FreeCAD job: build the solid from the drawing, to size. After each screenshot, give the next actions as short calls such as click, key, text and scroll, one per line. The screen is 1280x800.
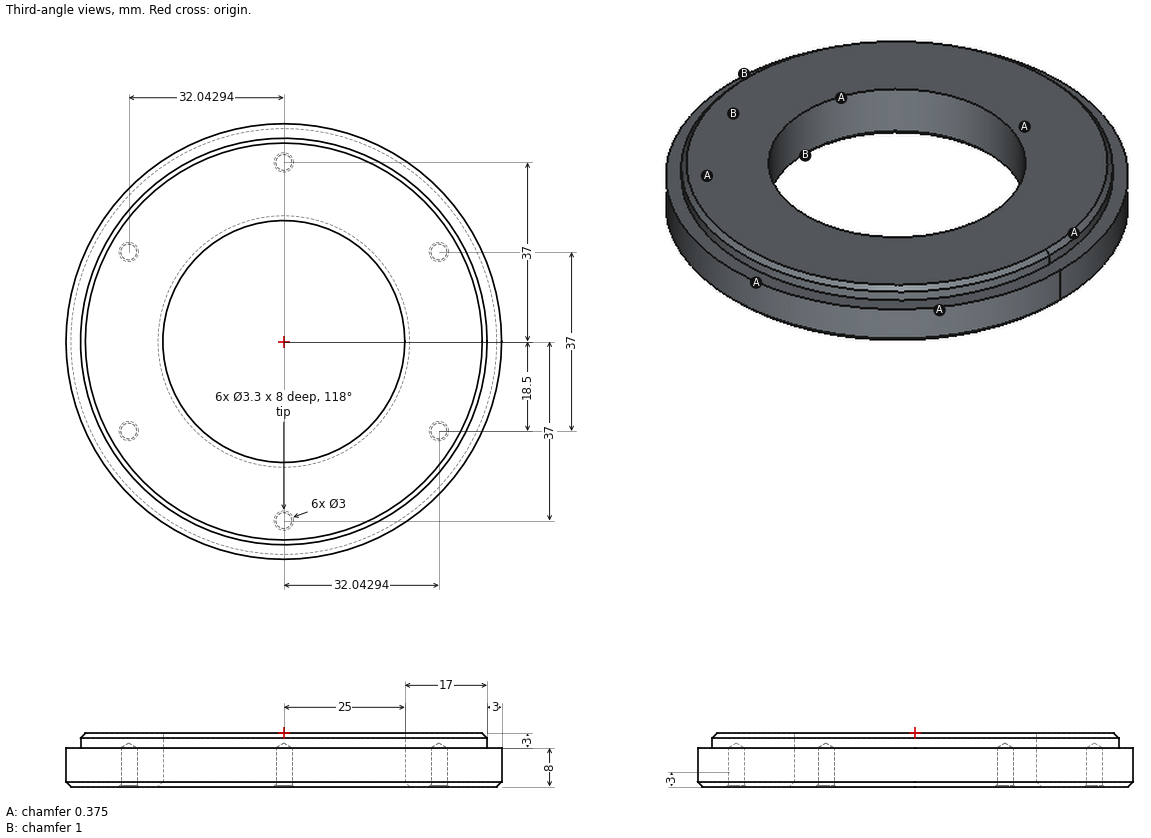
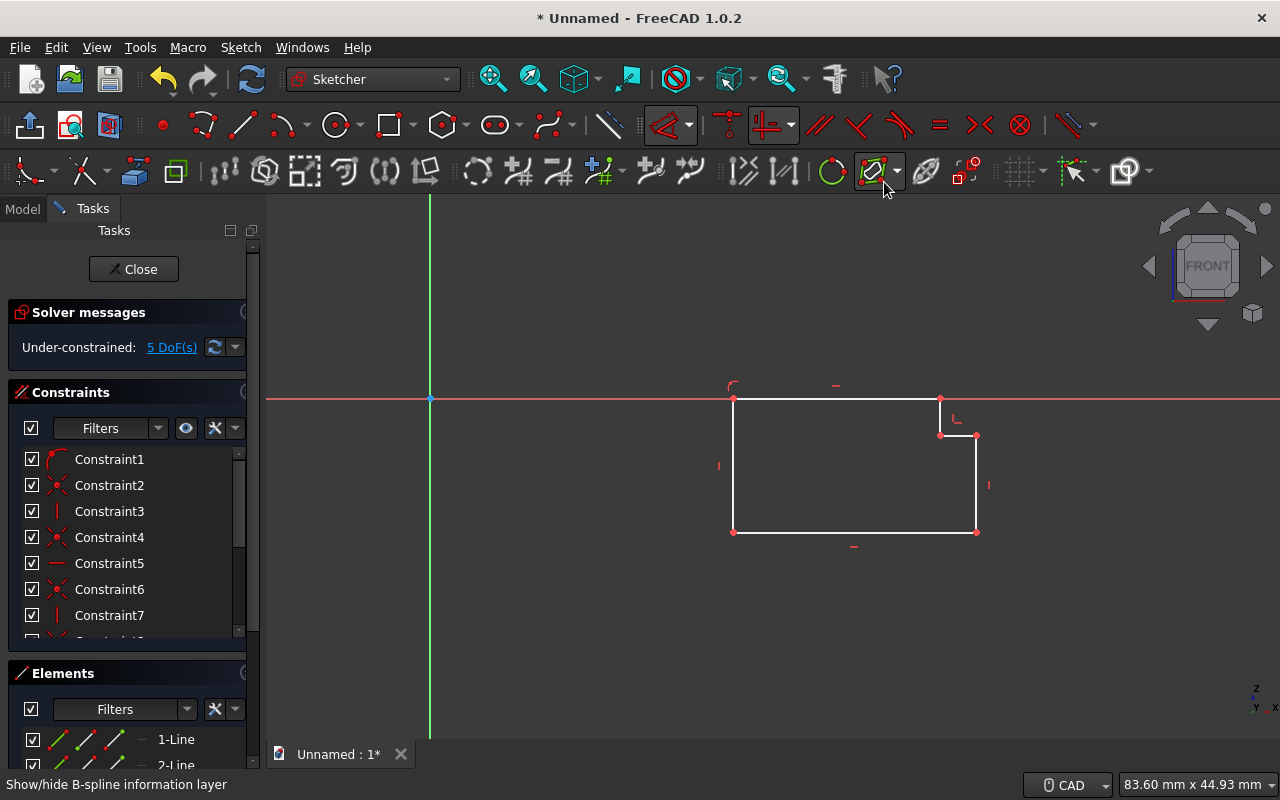
click(664, 126)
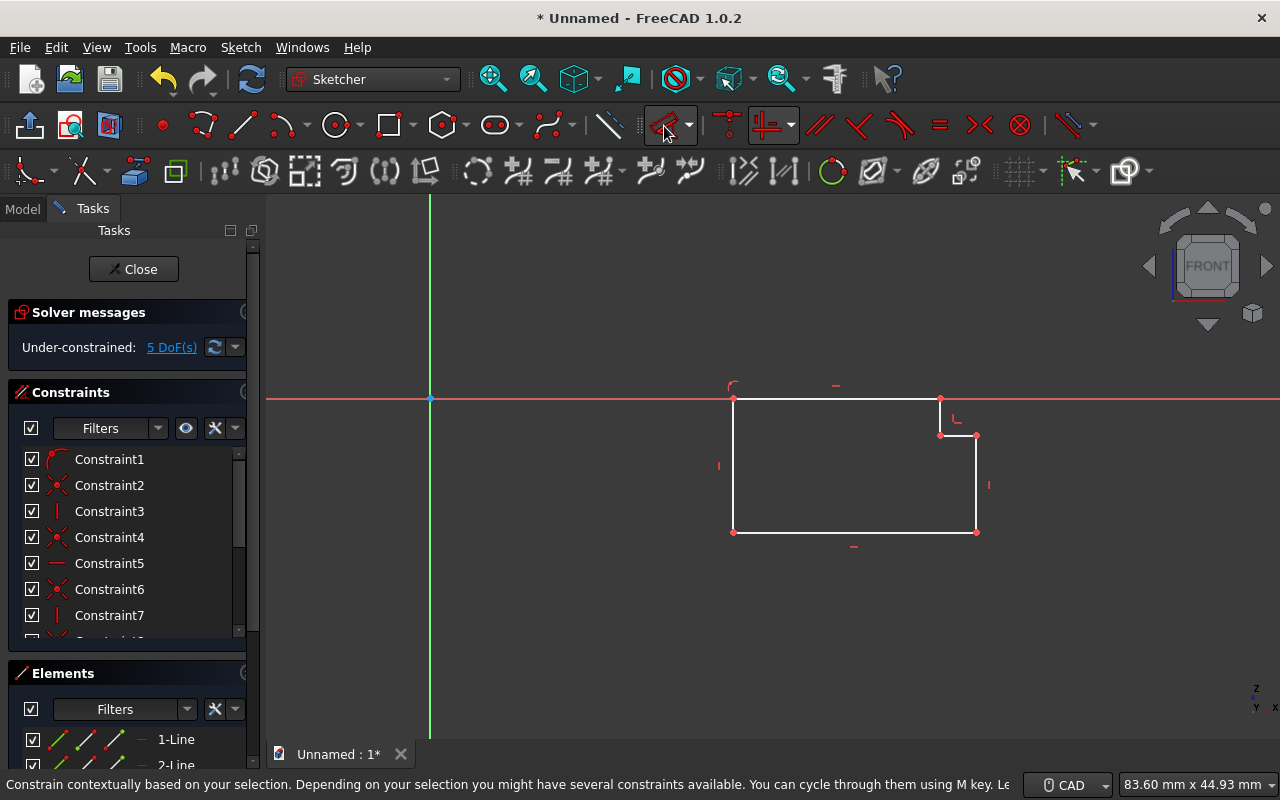
scroll(940, 410, up, 2)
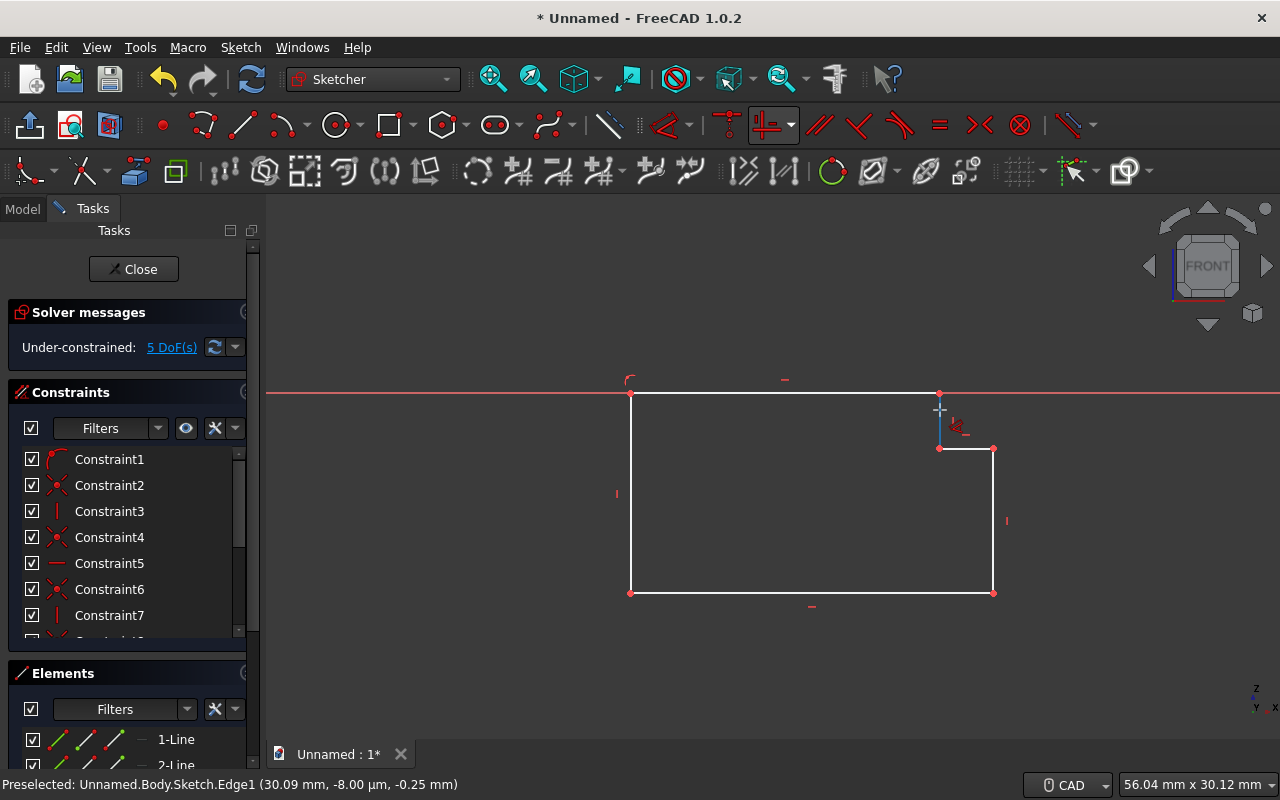
click(940, 410)
click(974, 421)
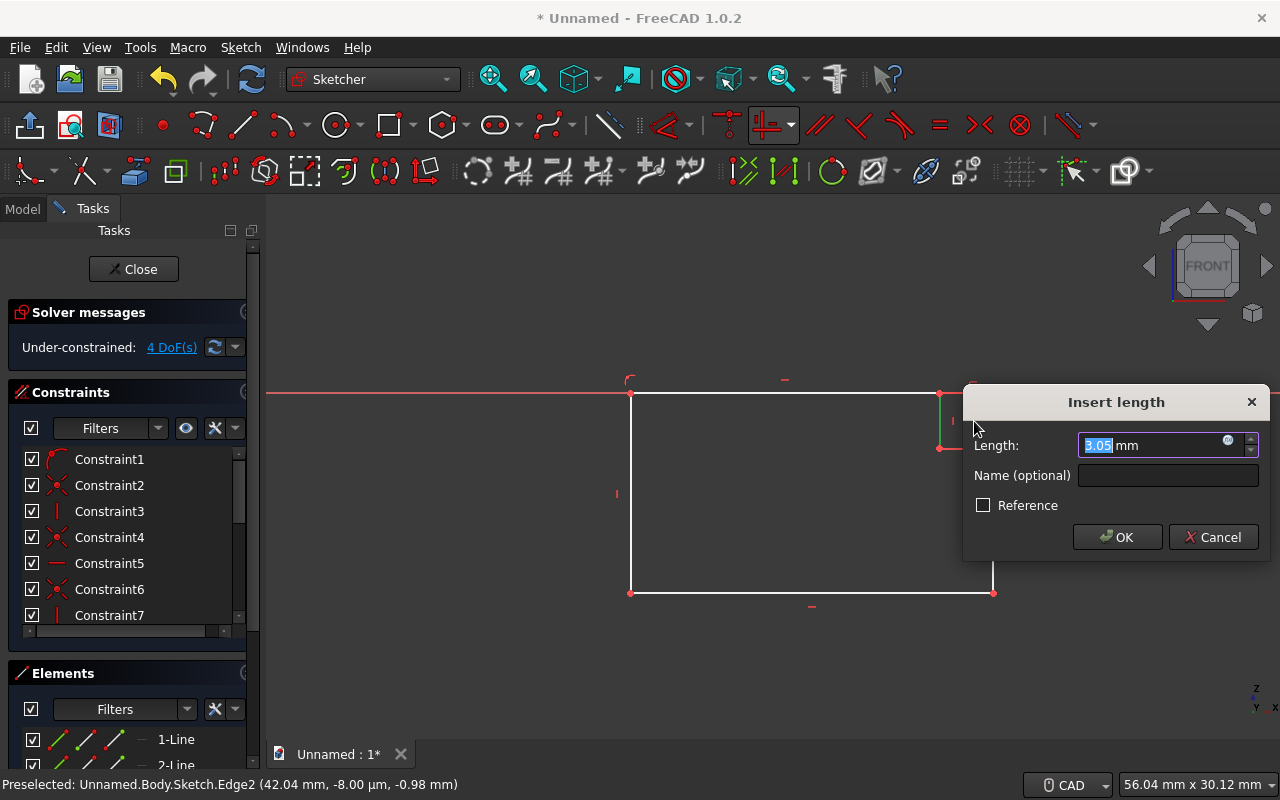
text(3)
key(Return)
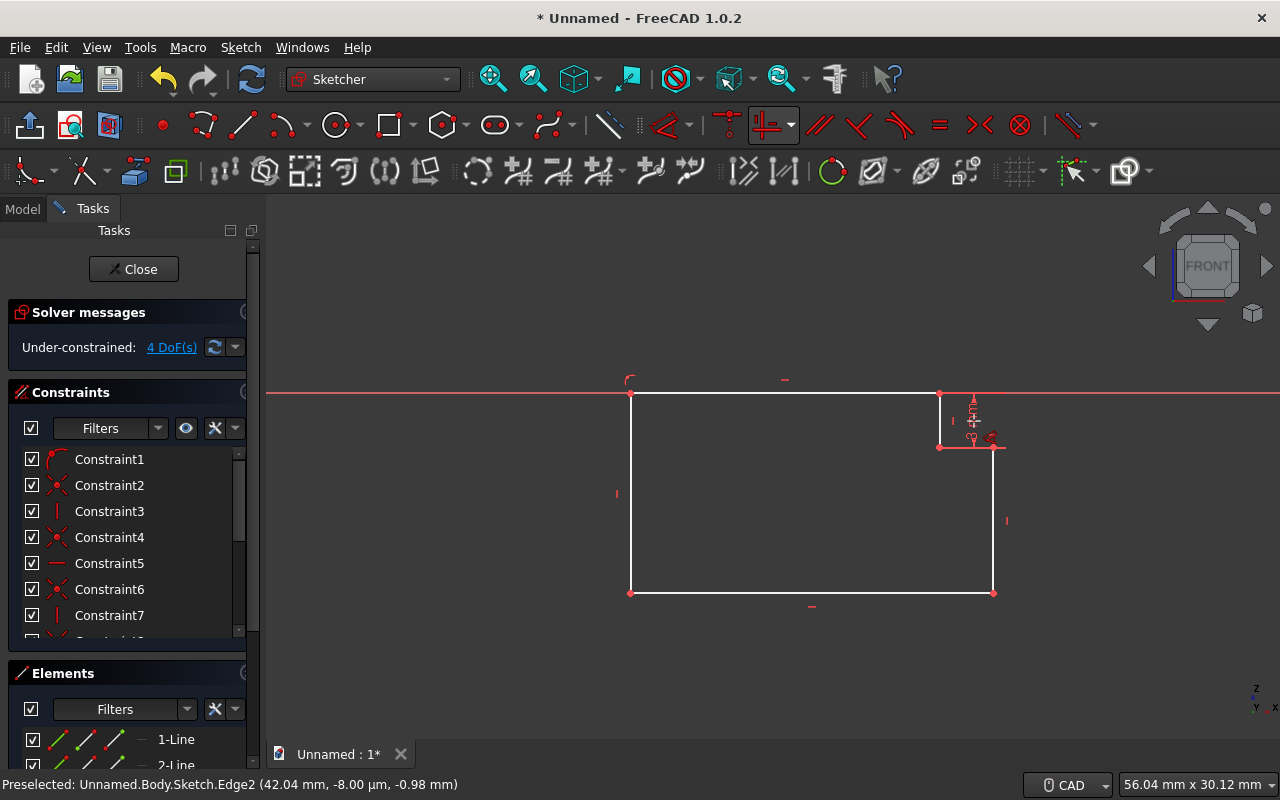
click(956, 448)
click(967, 482)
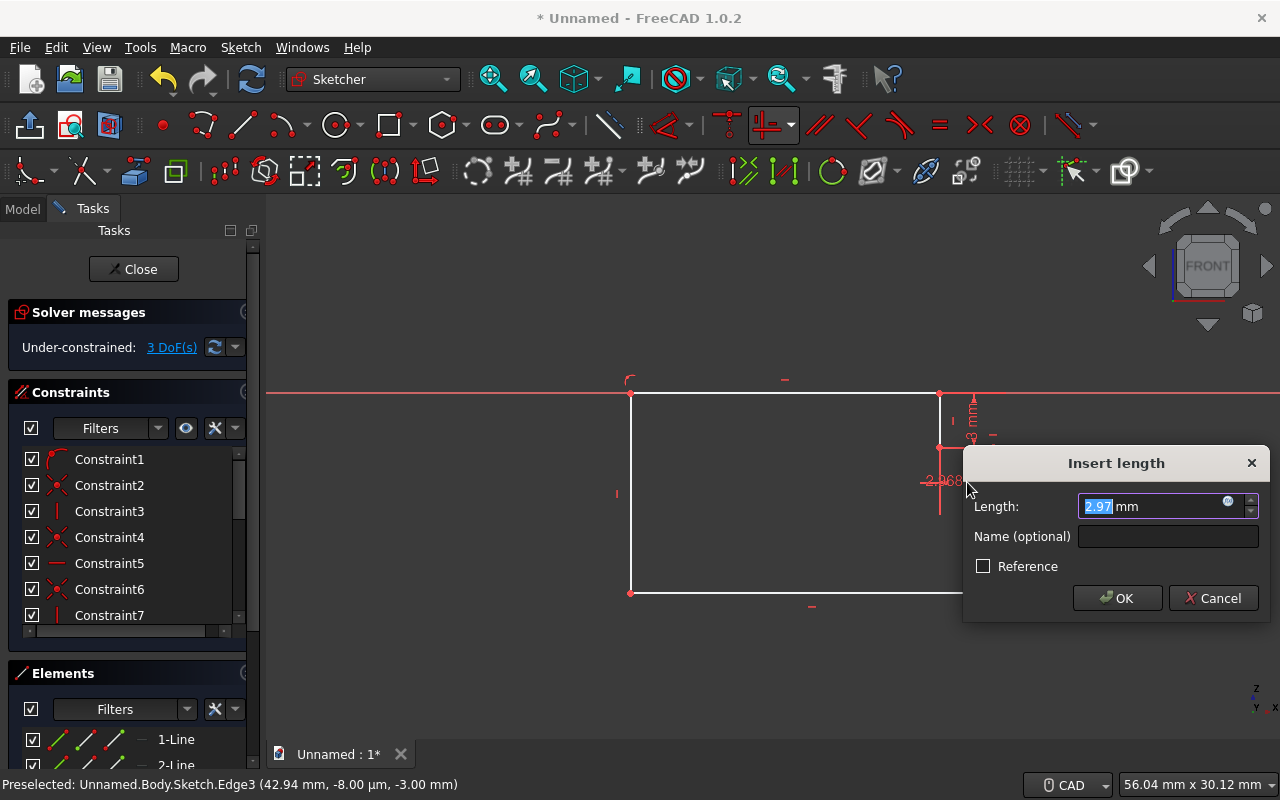
text(3)
key(Return)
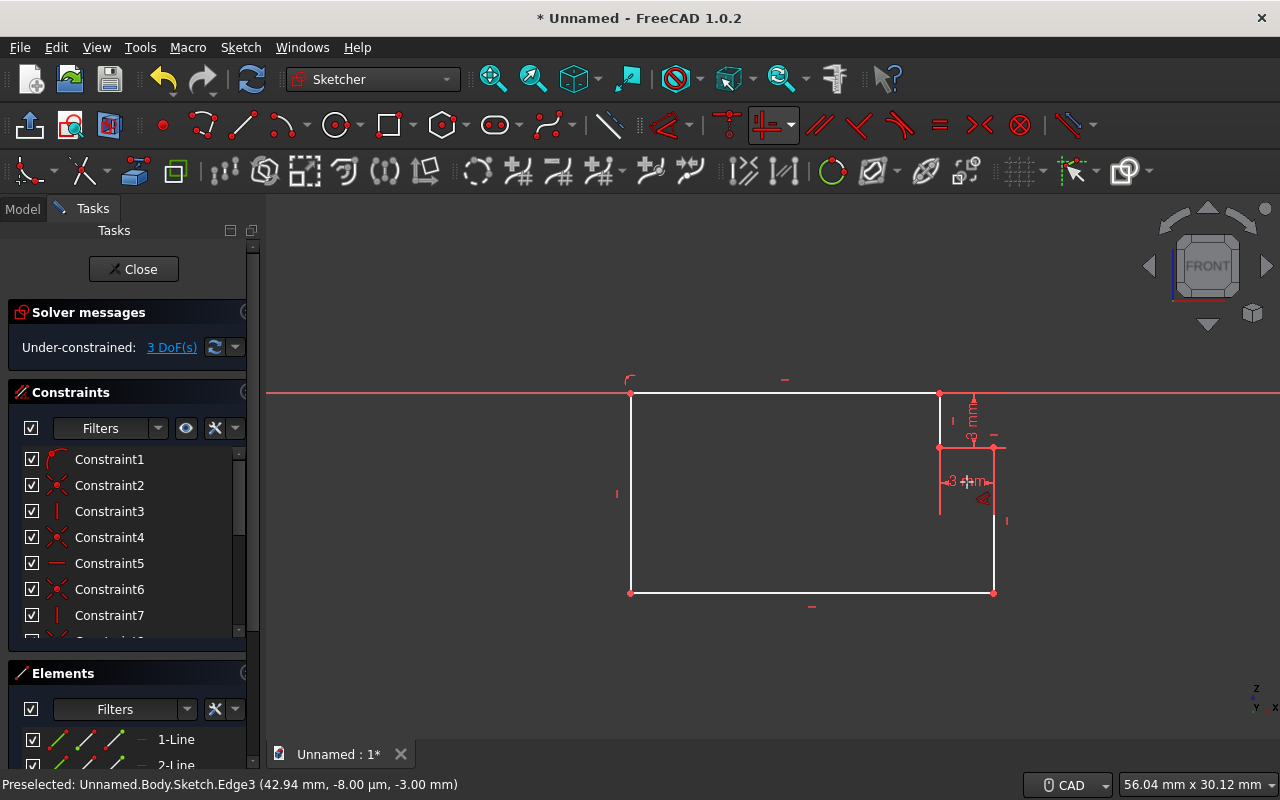
click(994, 491)
click(1028, 520)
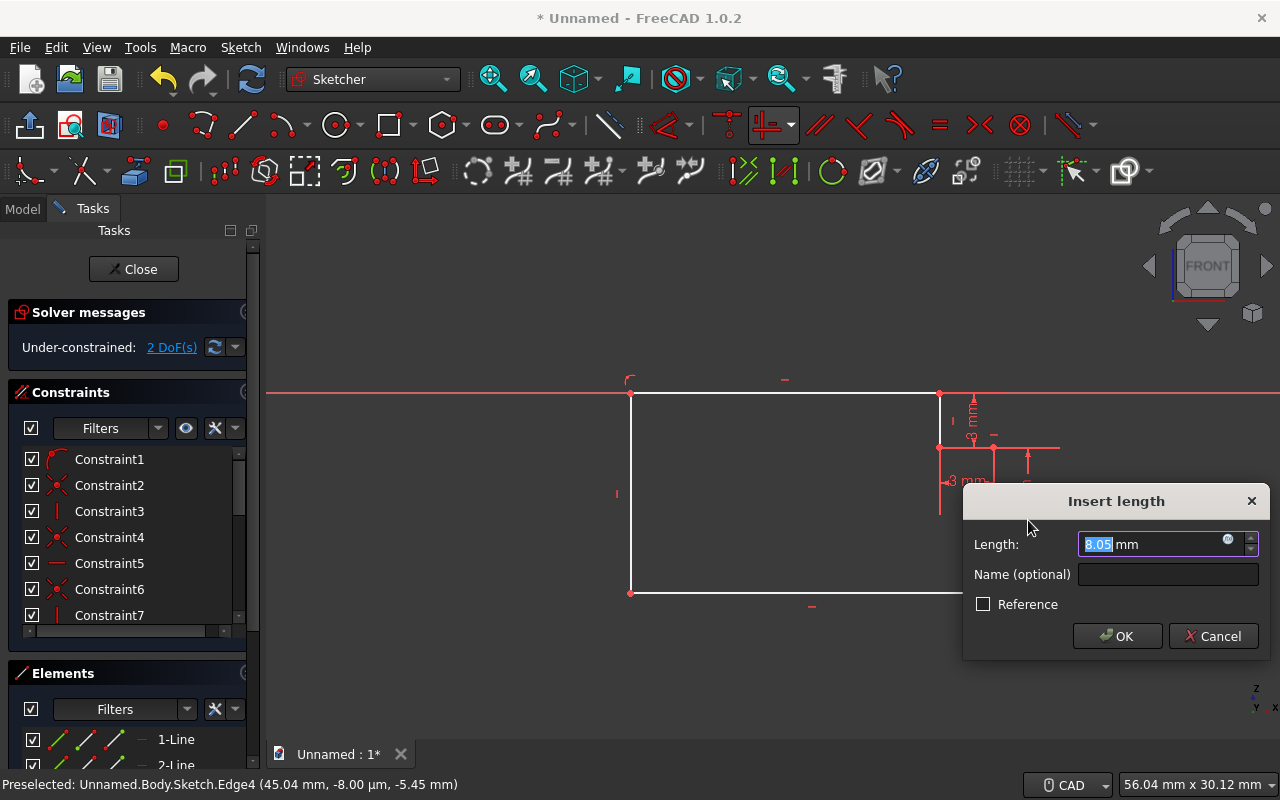
text(8)
key(Return)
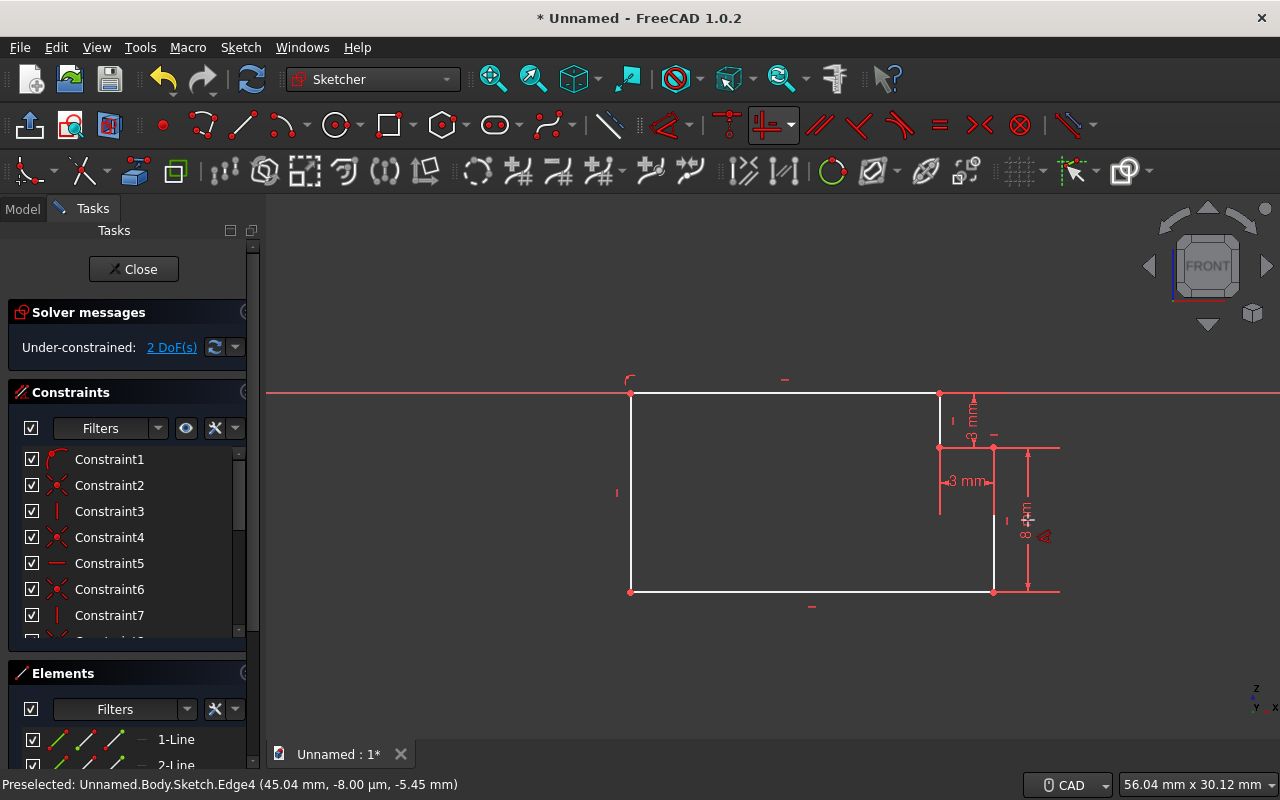
click(724, 393)
click(785, 359)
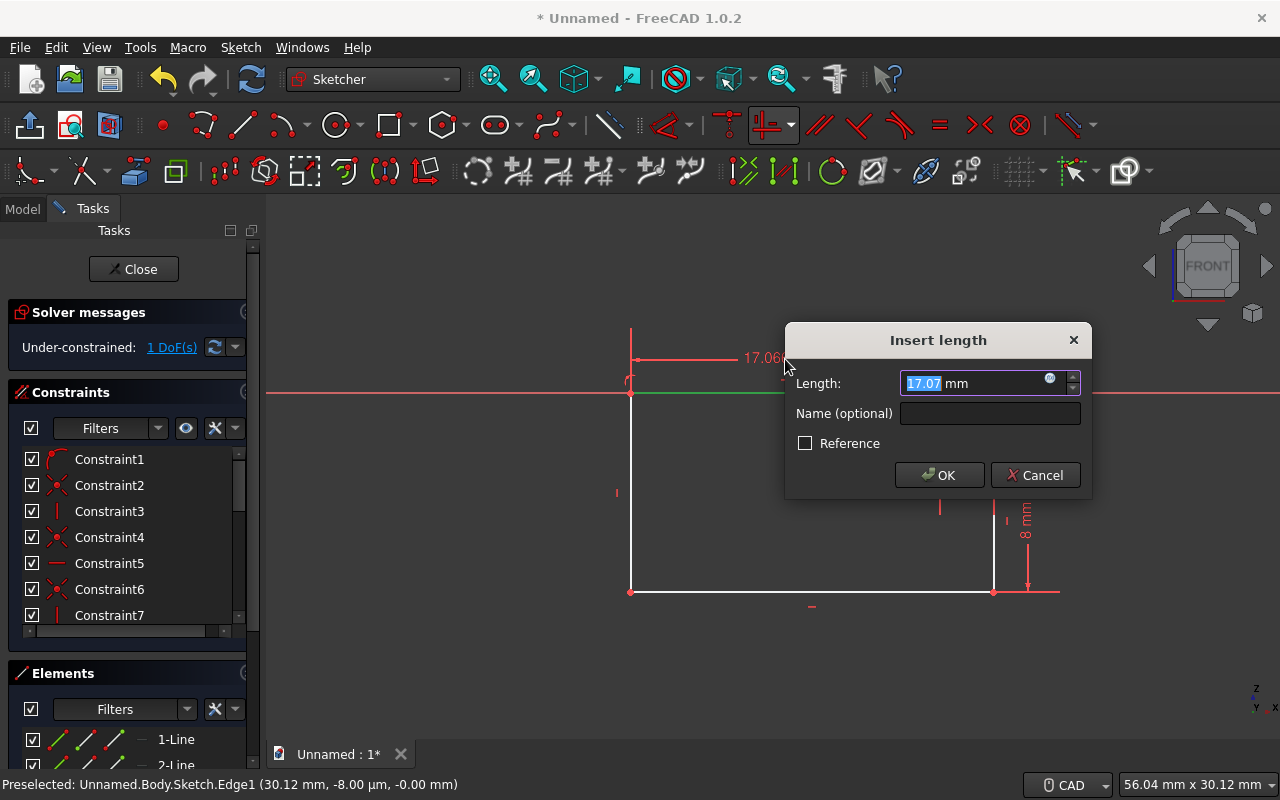
text(17)
key(Return)